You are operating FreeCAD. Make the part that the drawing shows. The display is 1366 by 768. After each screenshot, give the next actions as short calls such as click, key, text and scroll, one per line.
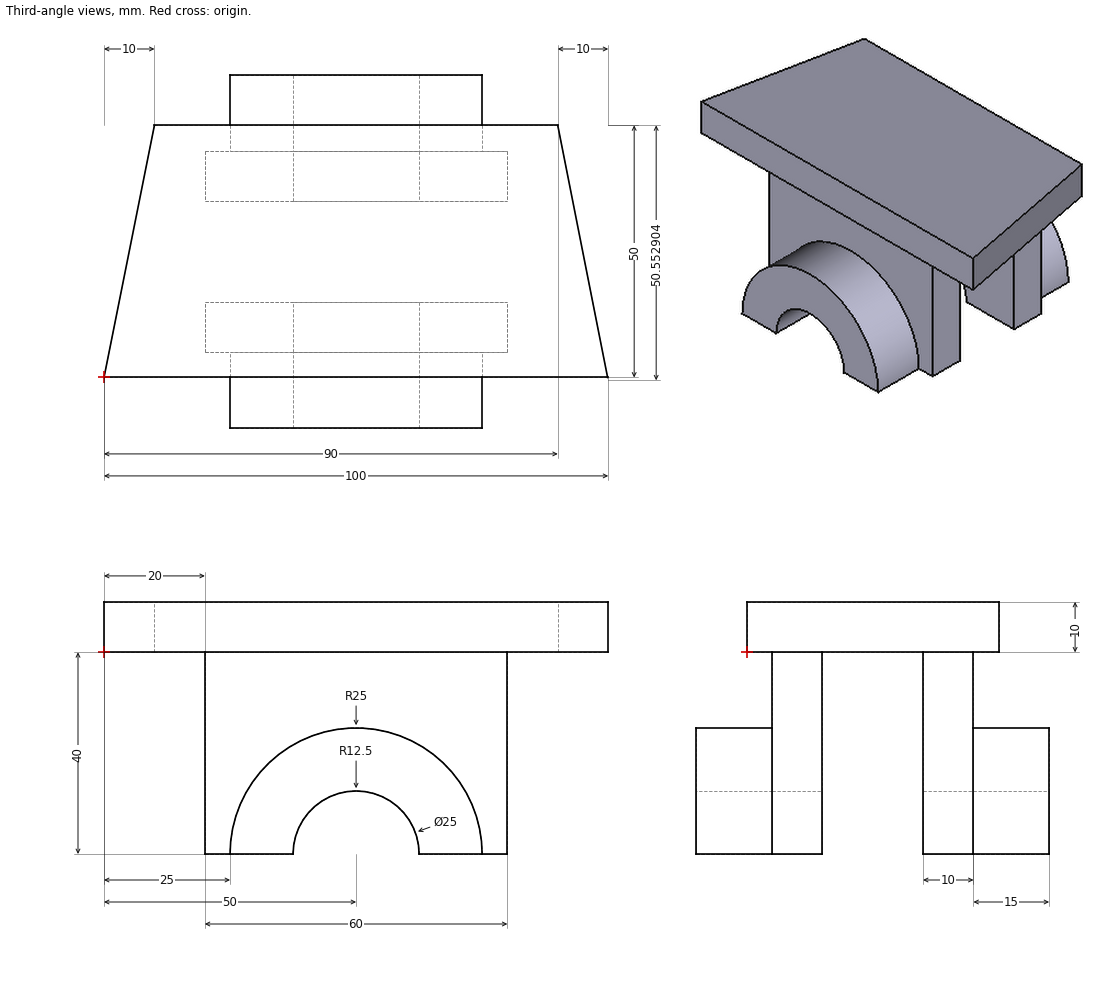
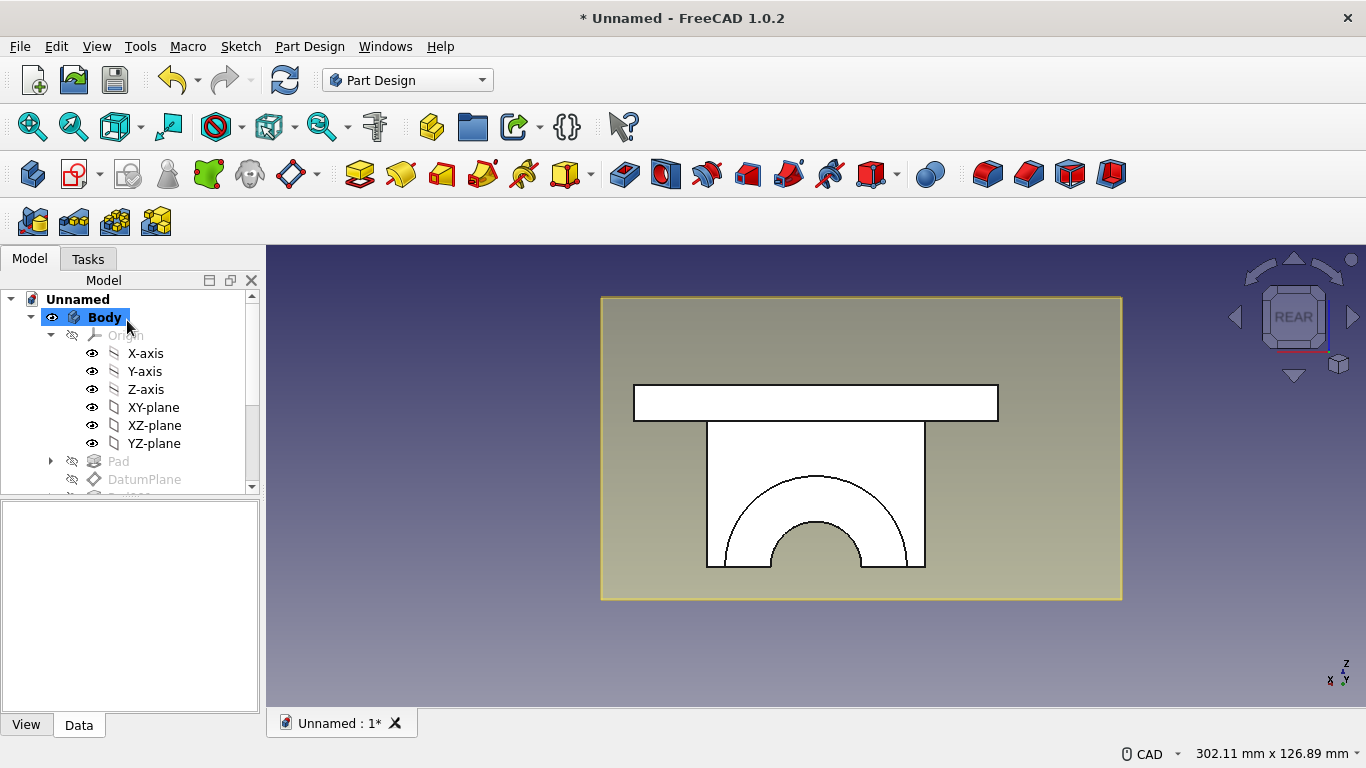
scroll(101, 385, down, 3)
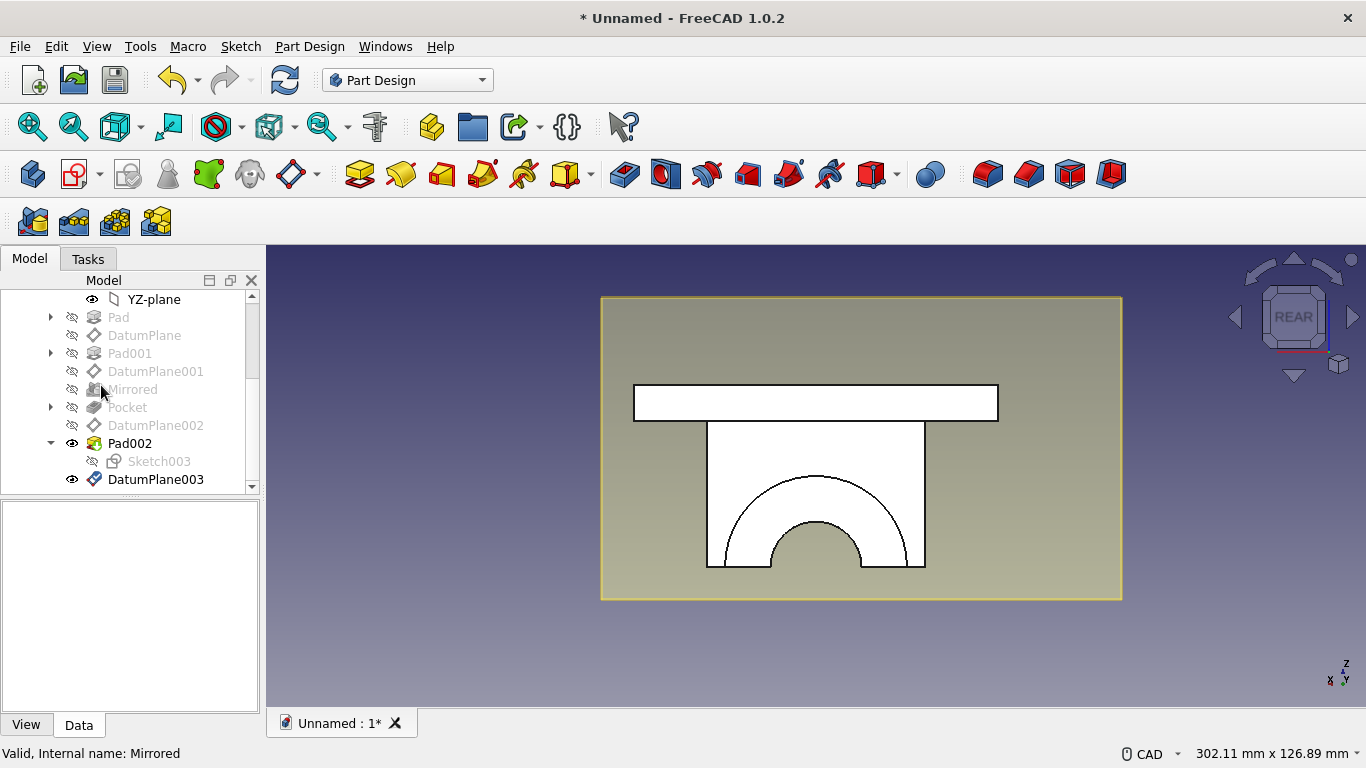
click(117, 443)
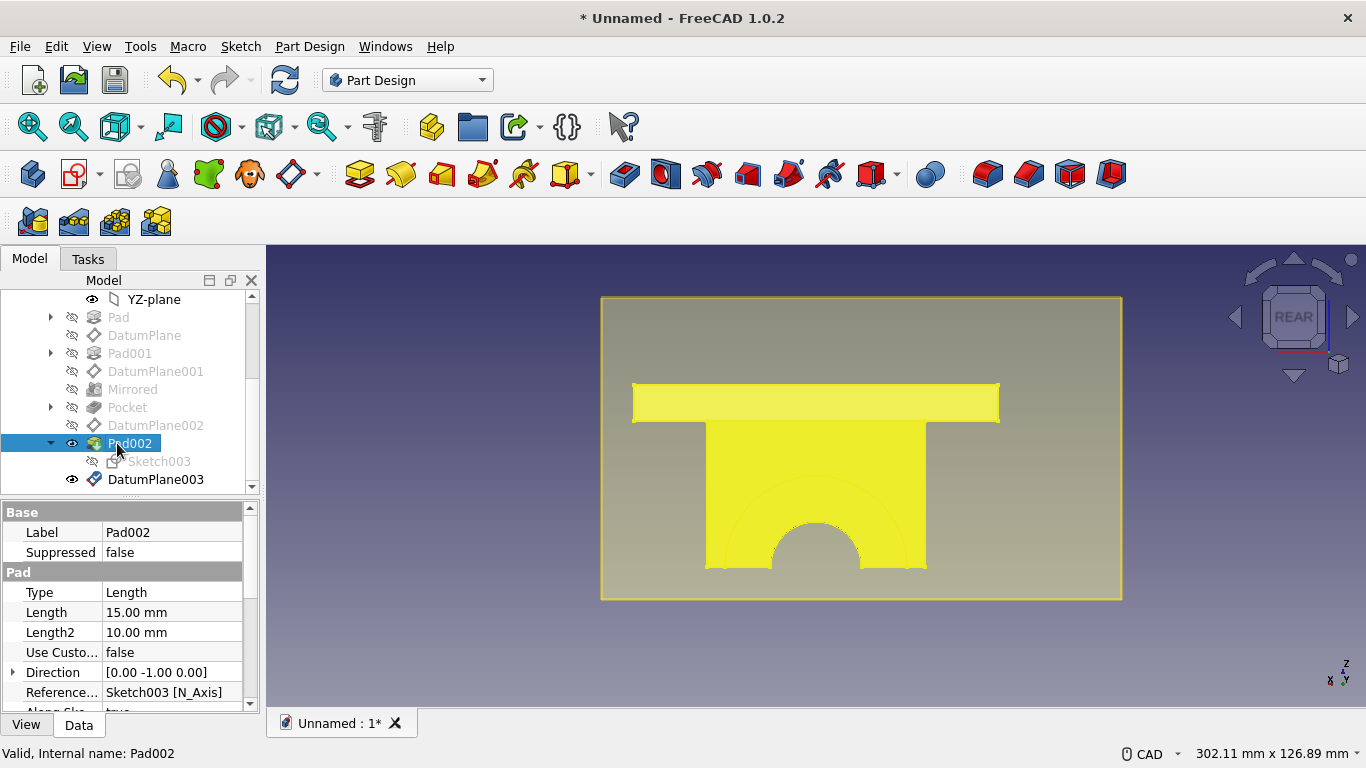
click(33, 222)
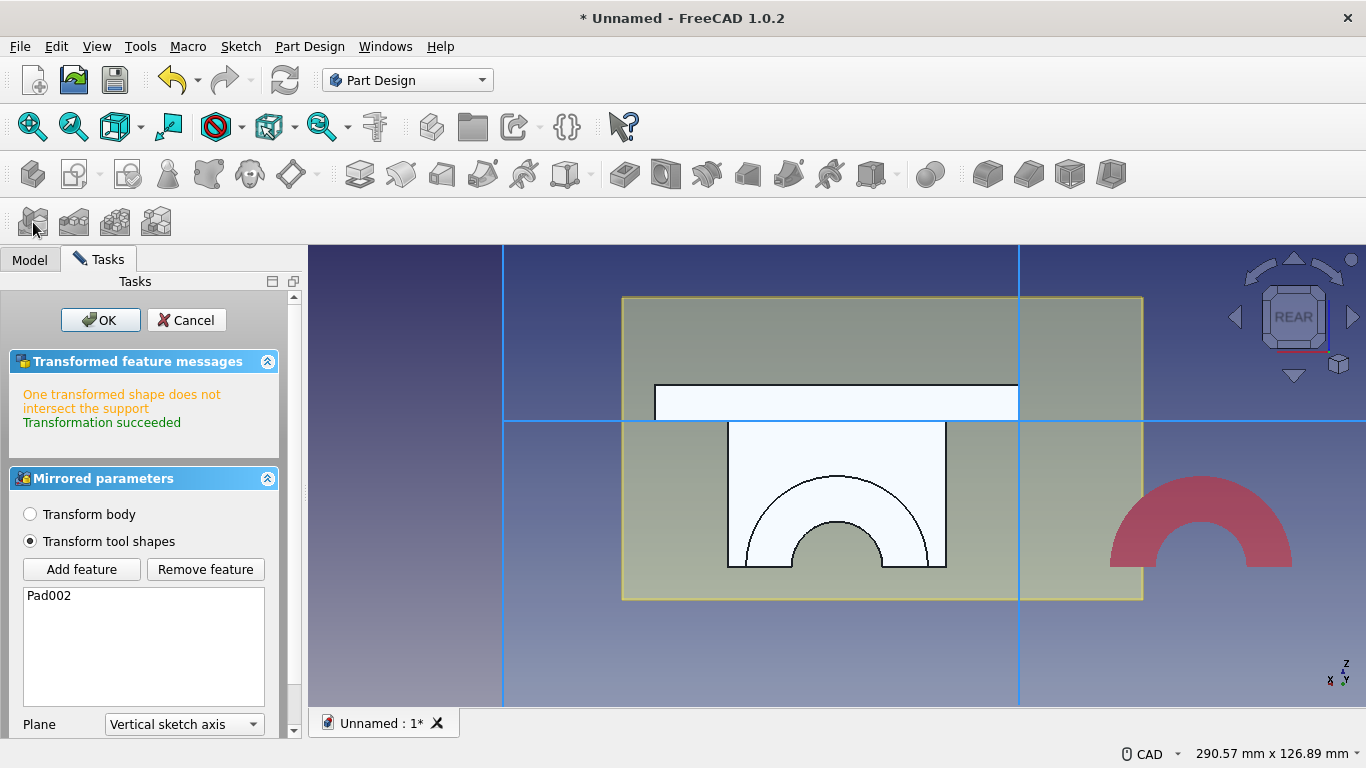
click(185, 724)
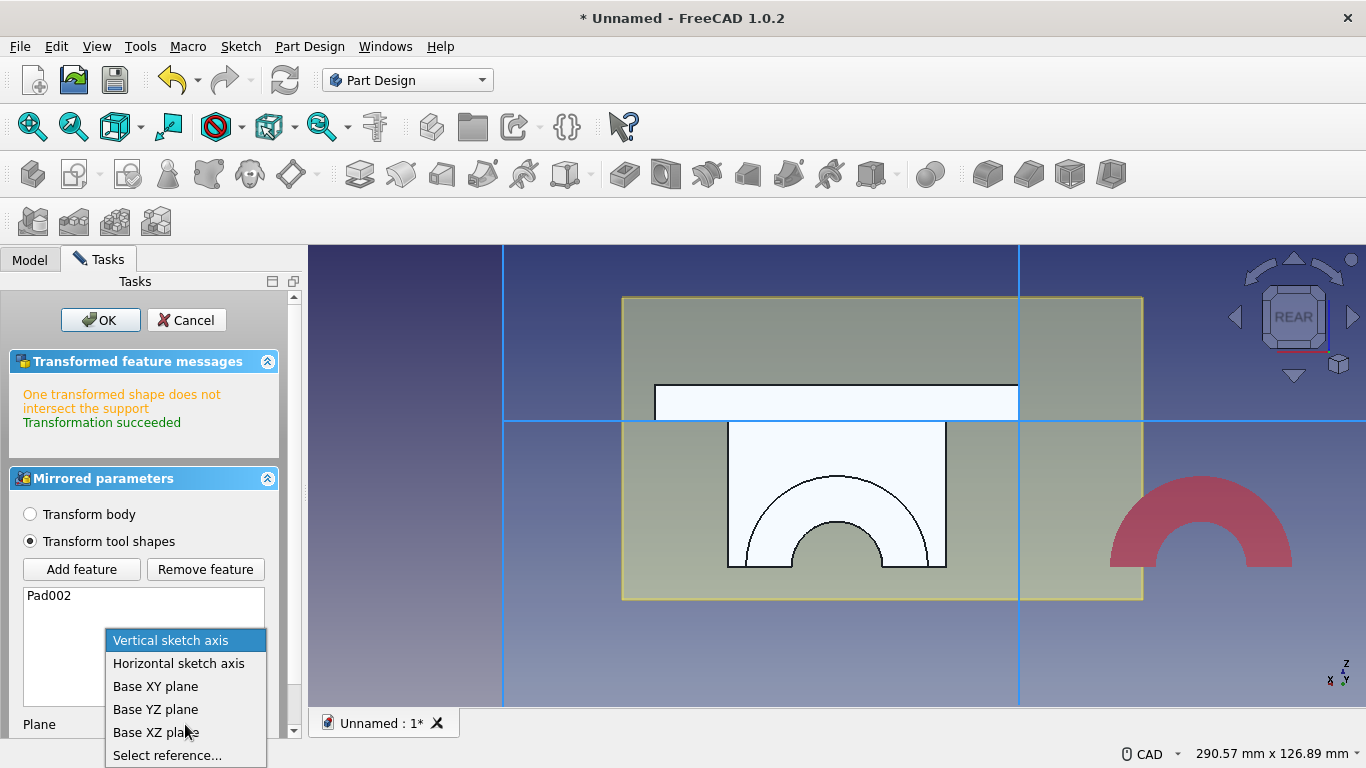
click(184, 756)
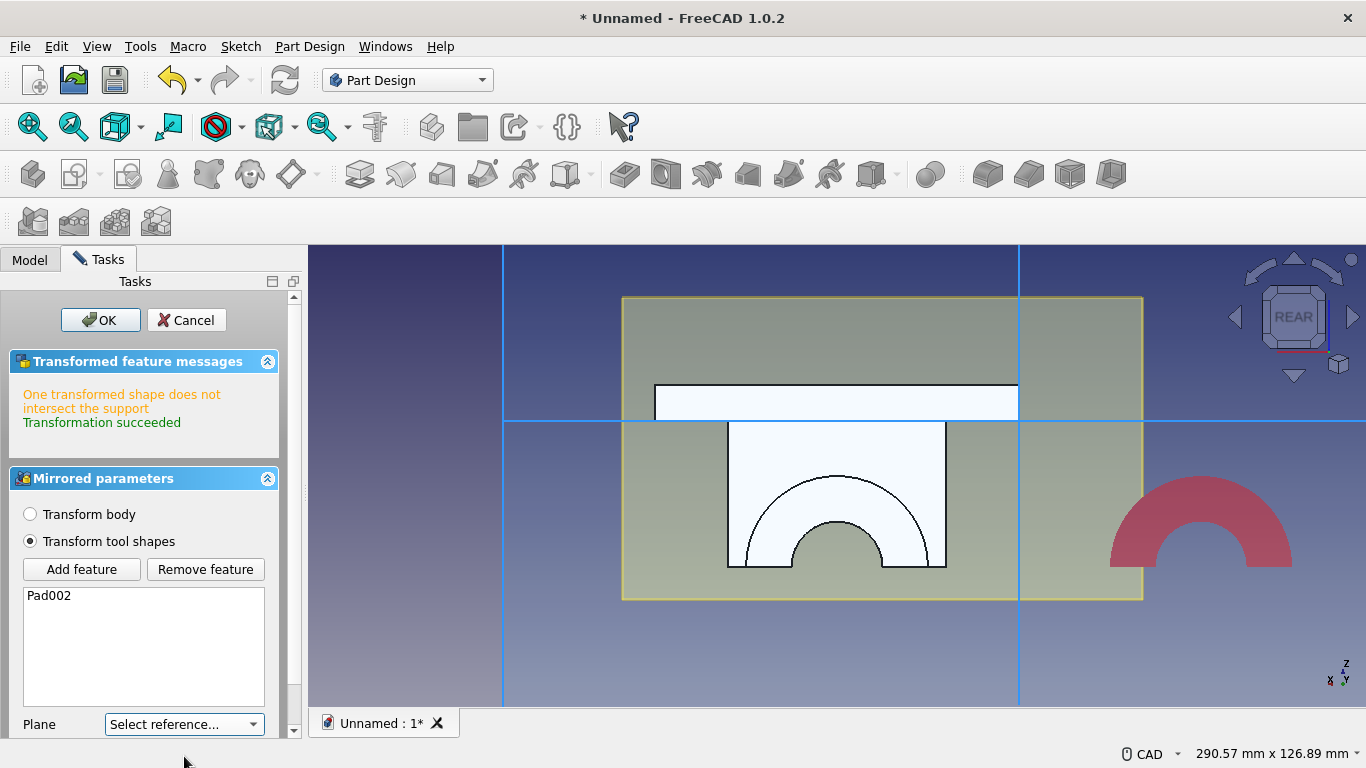
click(30, 259)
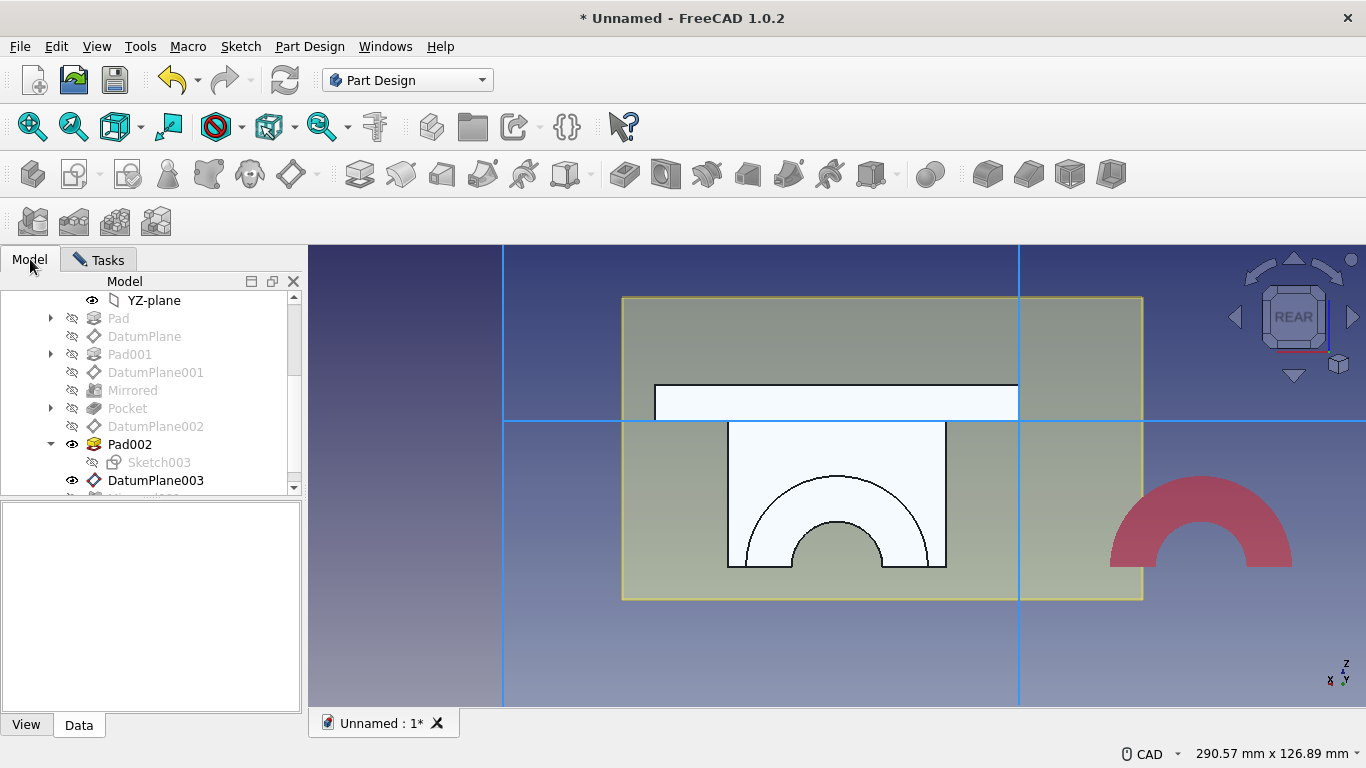
click(117, 480)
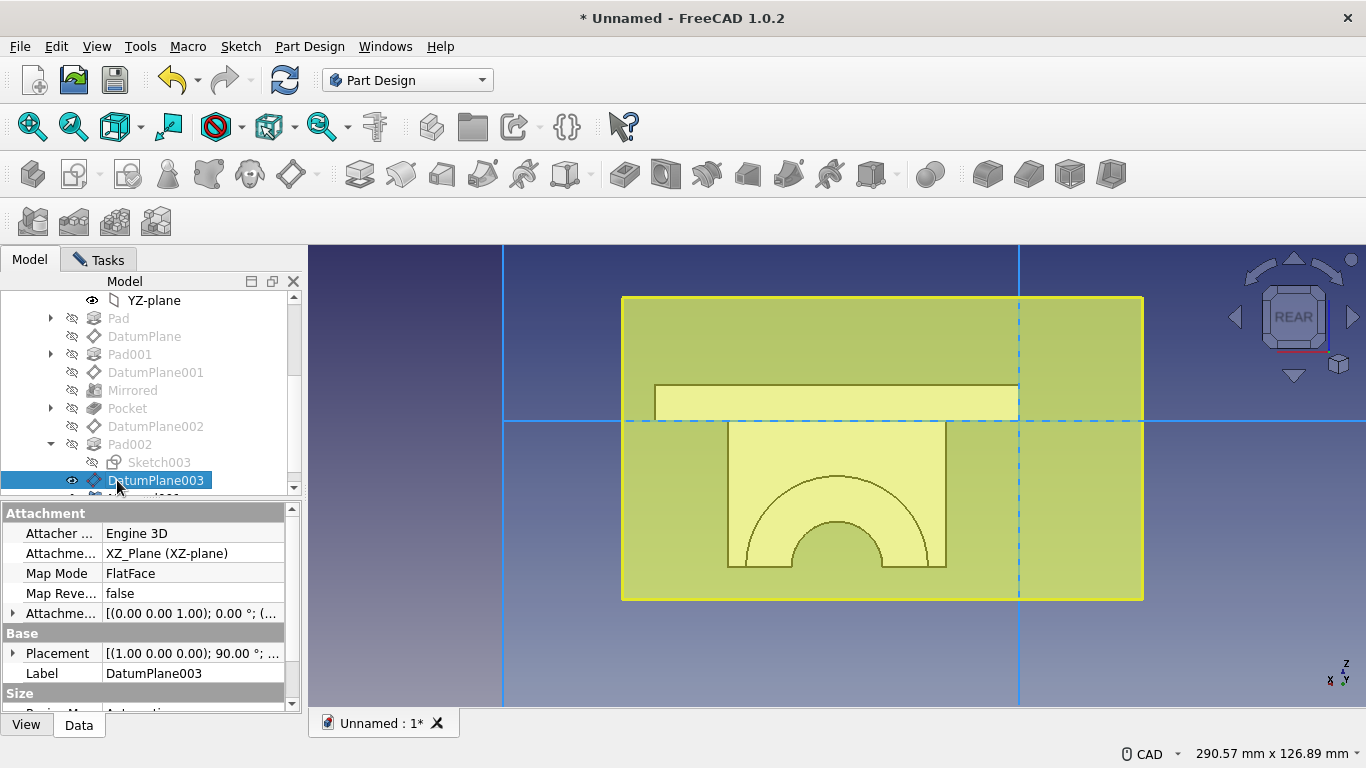
click(98, 259)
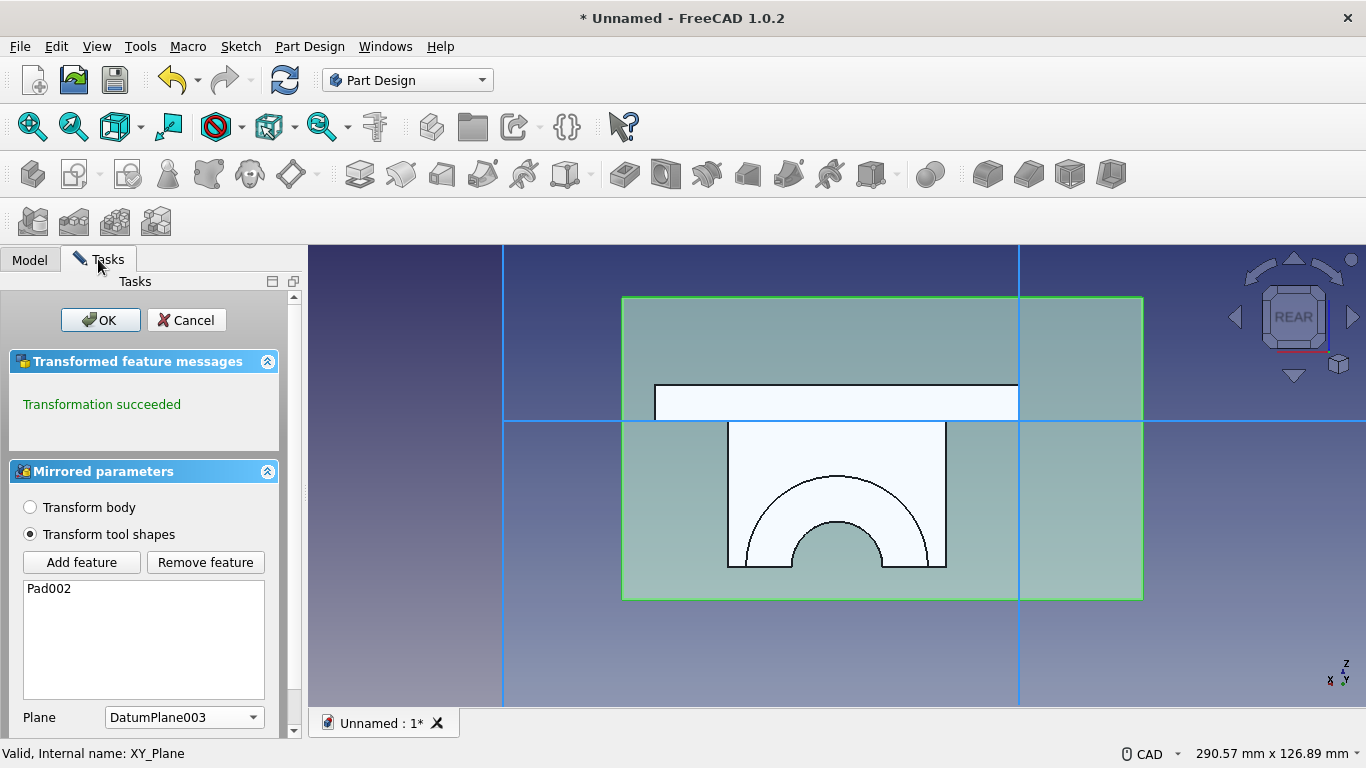
click(101, 320)